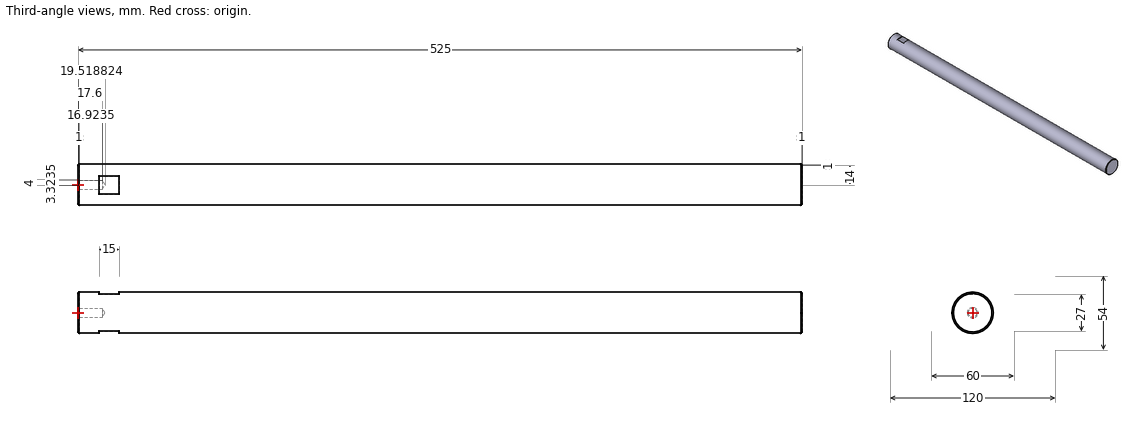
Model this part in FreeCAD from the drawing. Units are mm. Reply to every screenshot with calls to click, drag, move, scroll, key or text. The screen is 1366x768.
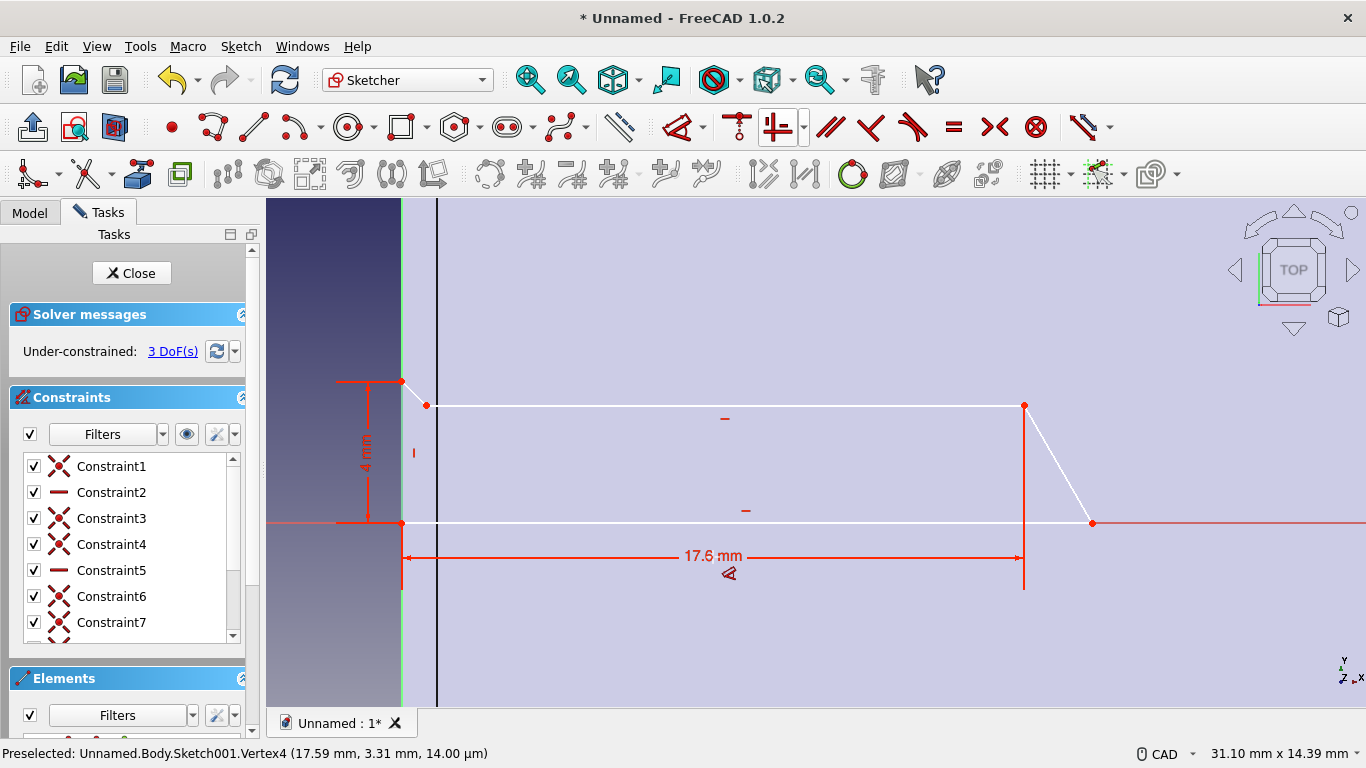
click(845, 406)
click(725, 372)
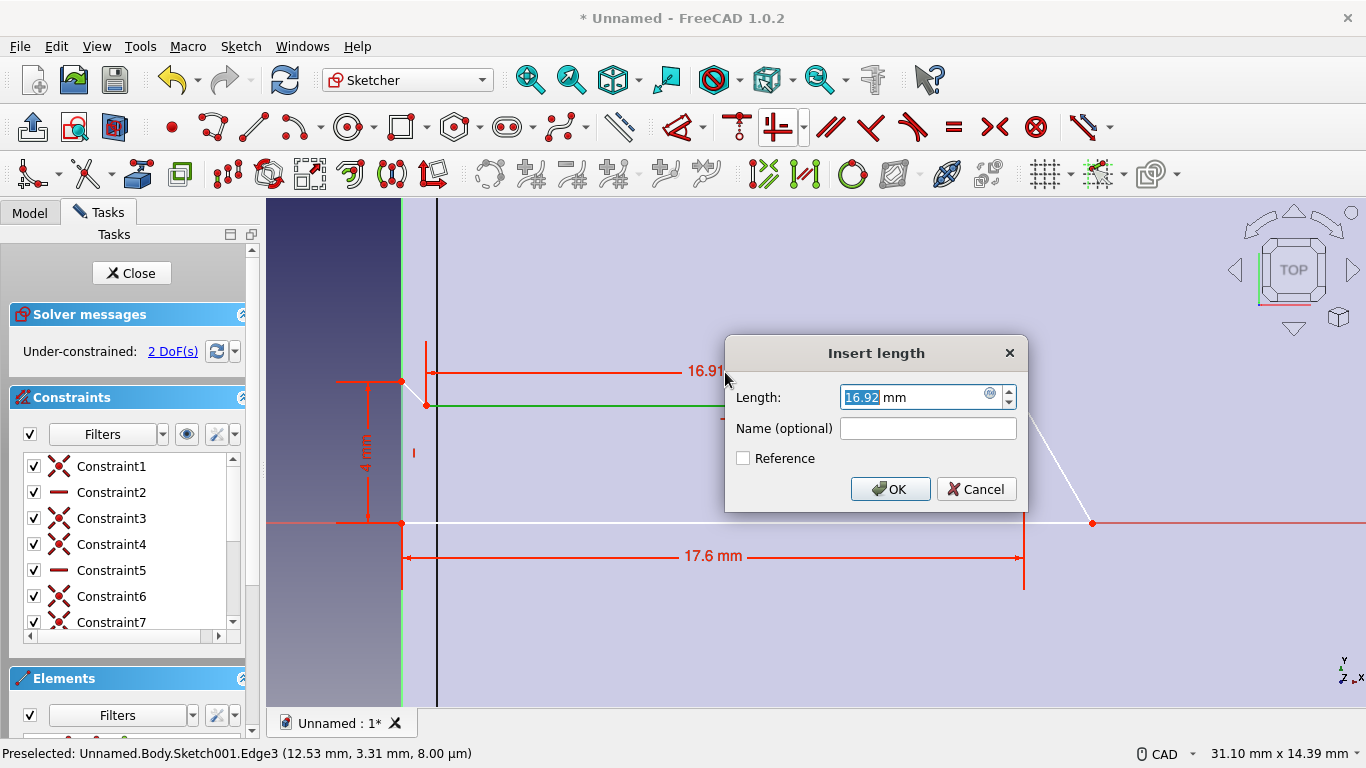
text(16.9235)
key(Return)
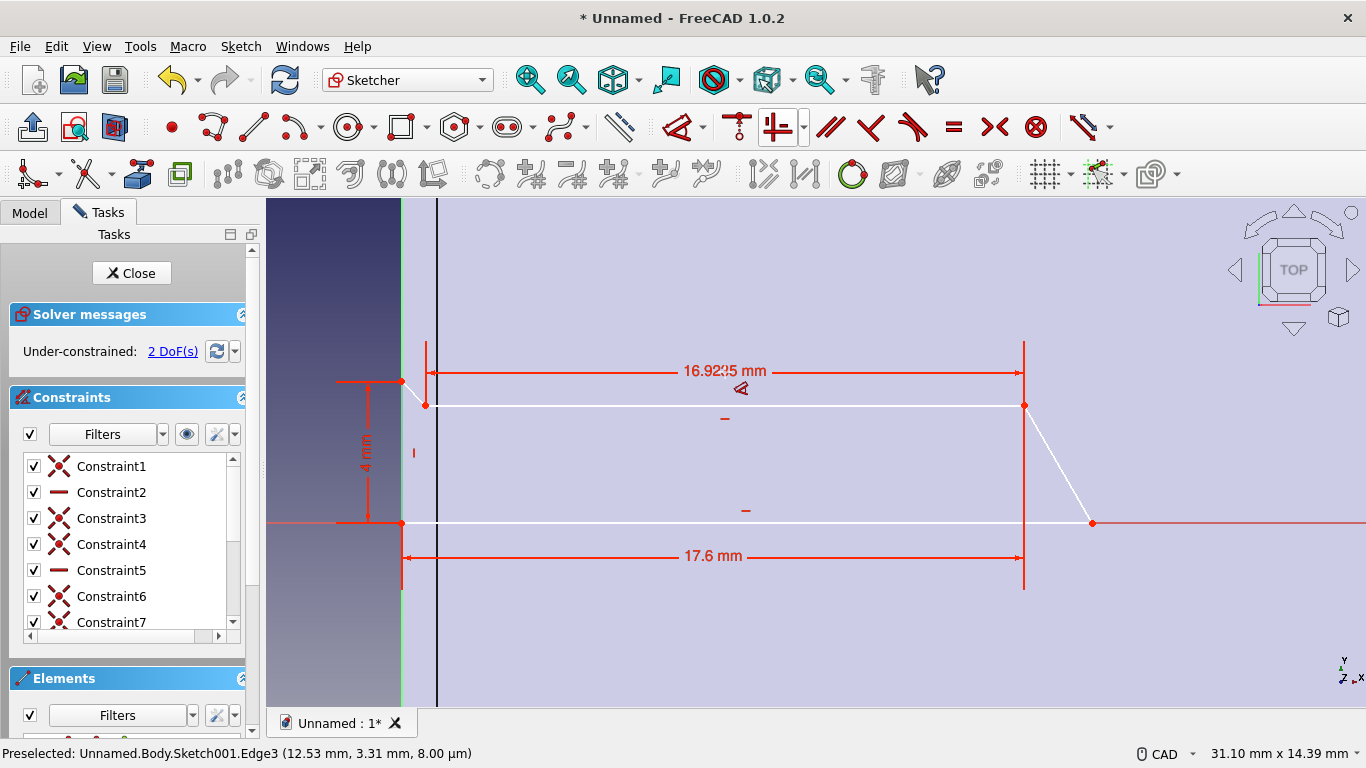
click(1024, 406)
click(368, 491)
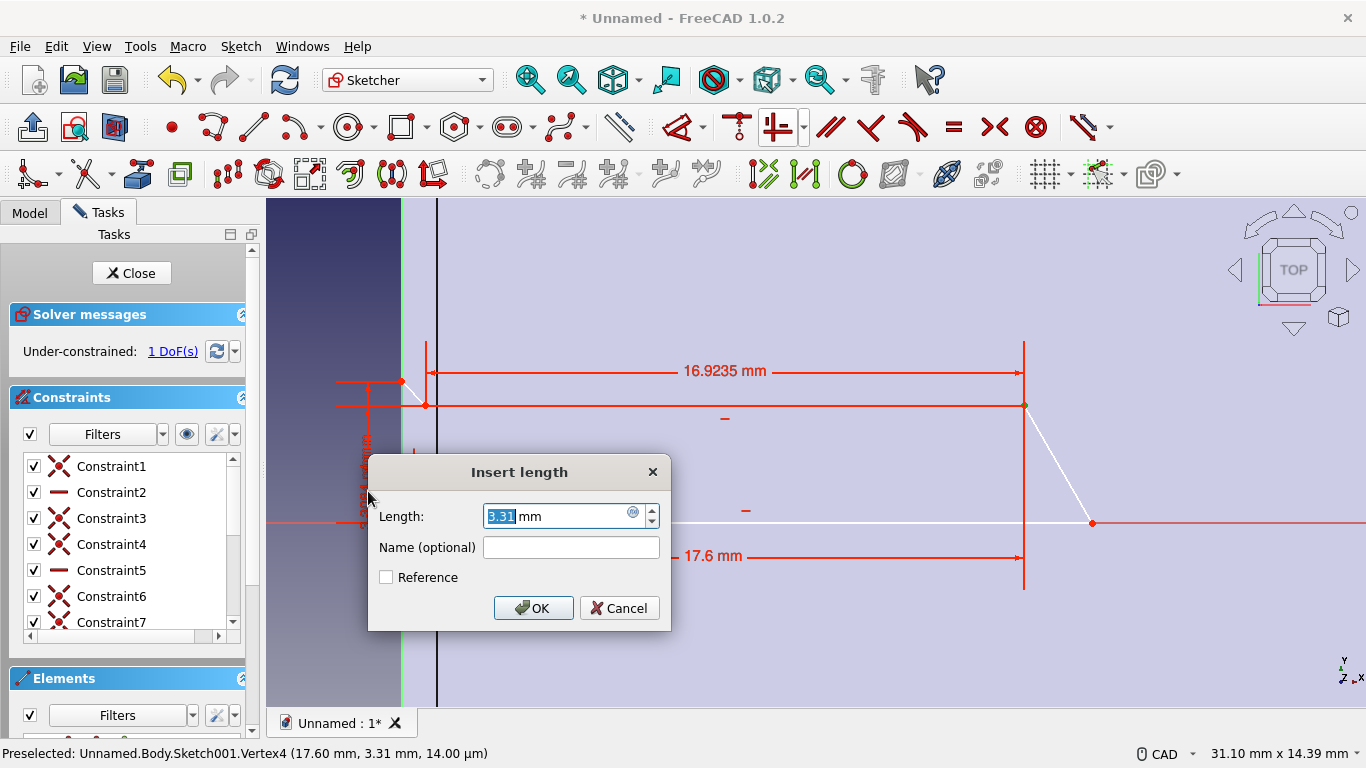
text(3.3235)
key(Return)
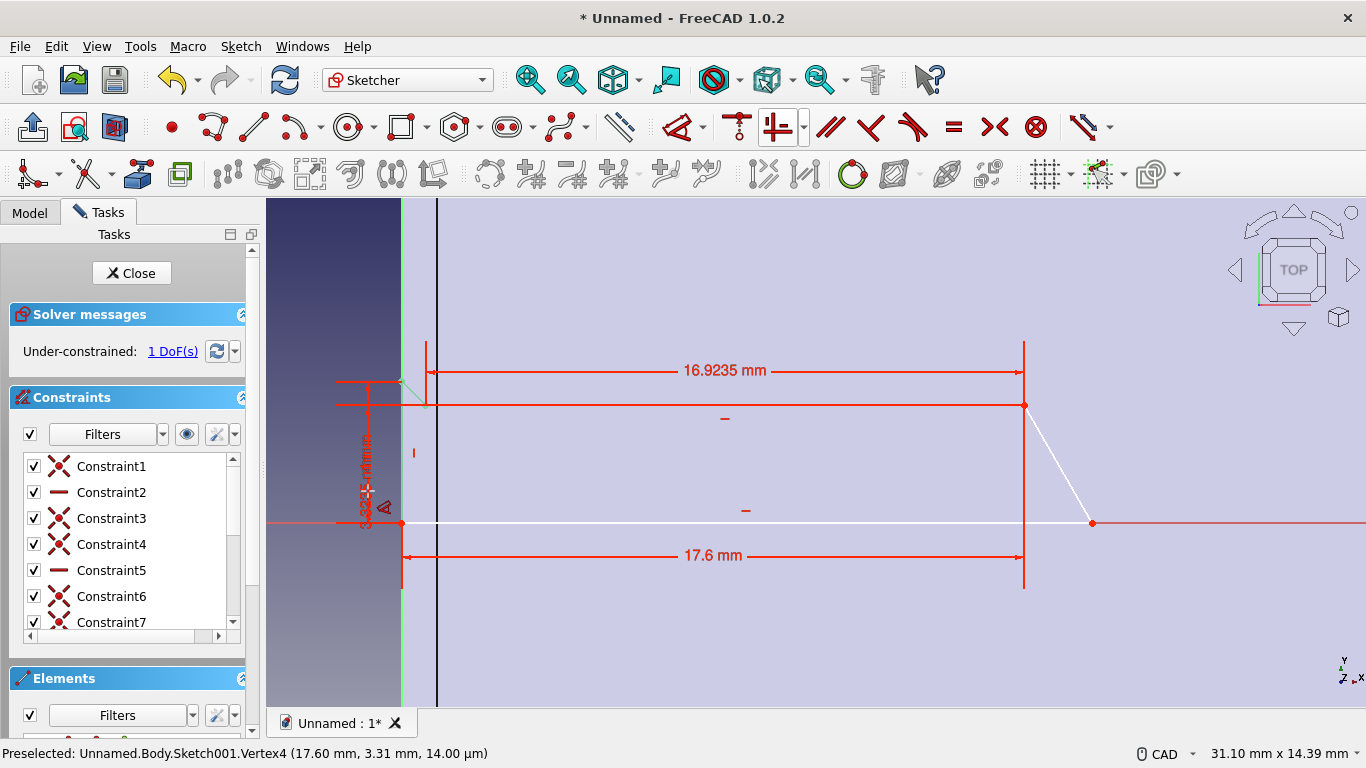
click(609, 523)
click(588, 557)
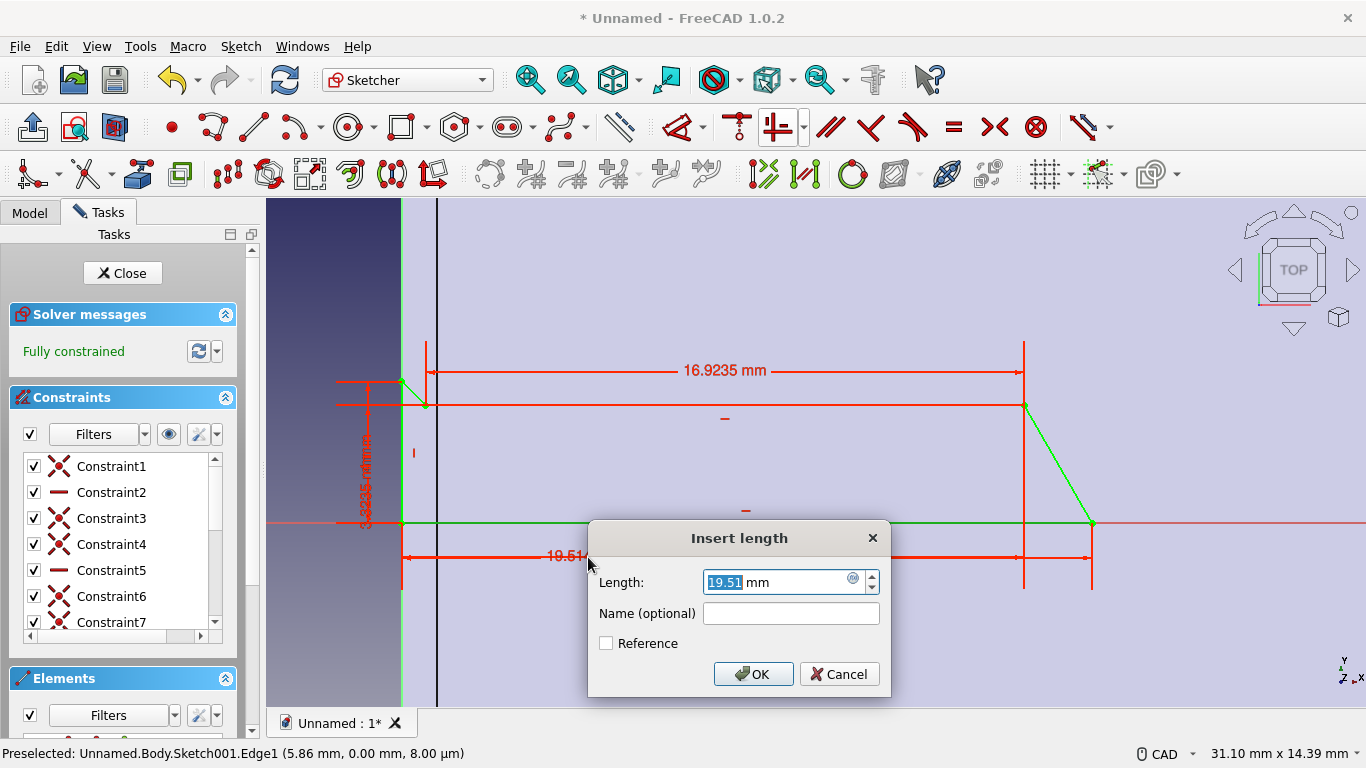
text(19.518824)
key(Return)
key(Escape)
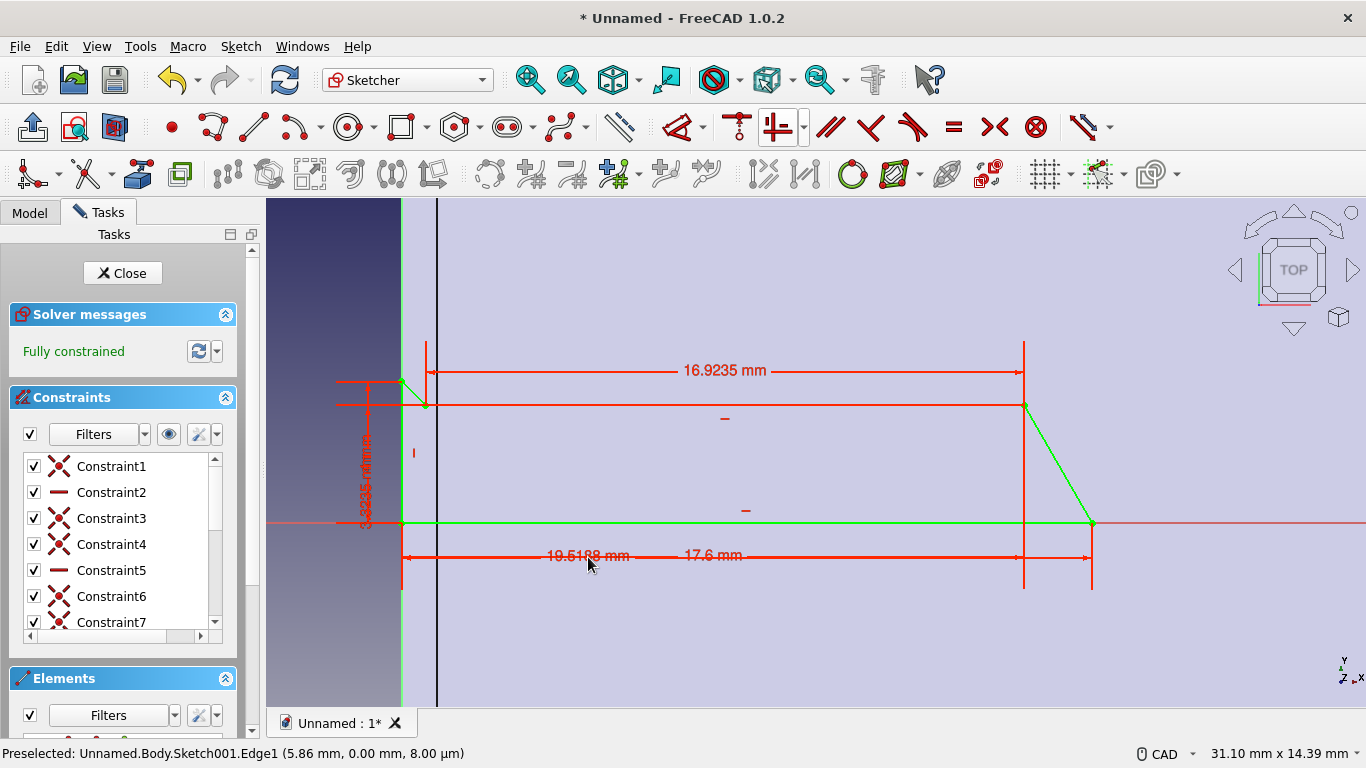
click(123, 273)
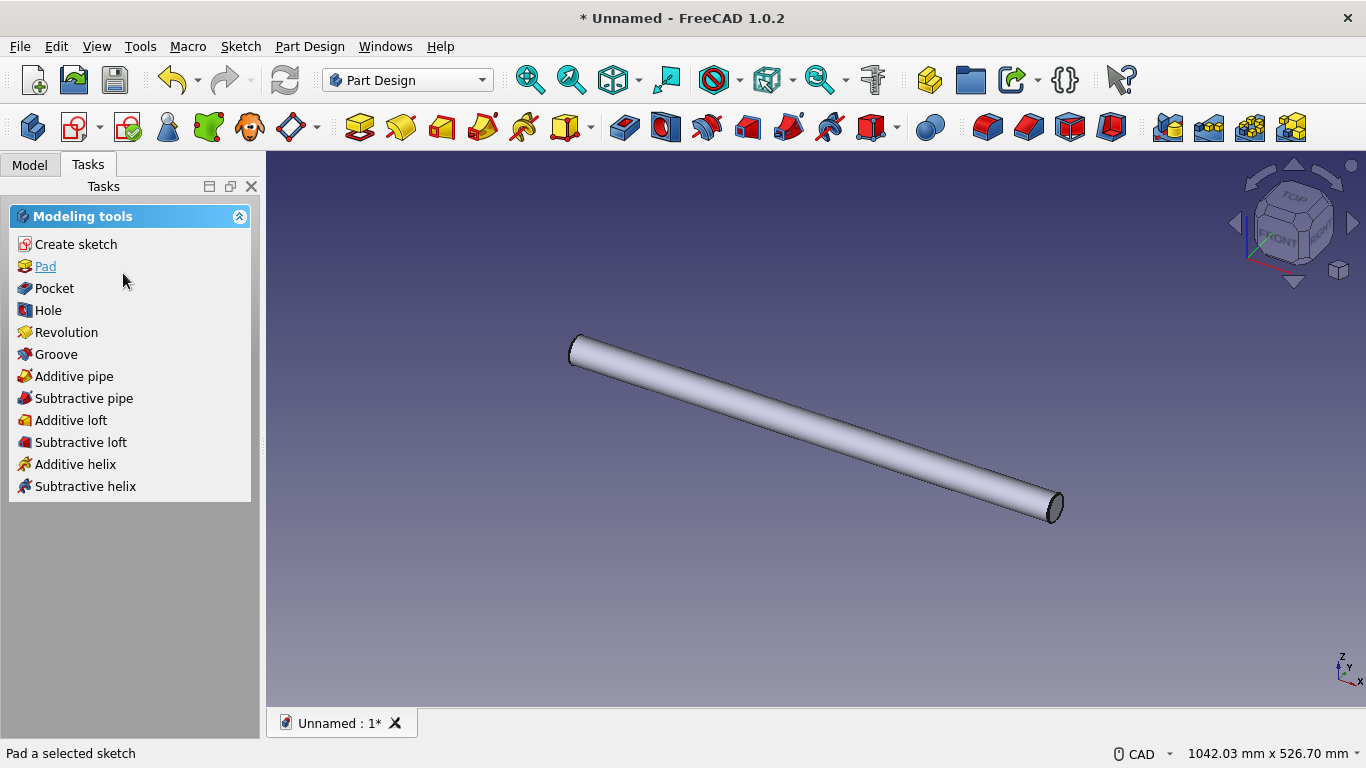
click(707, 128)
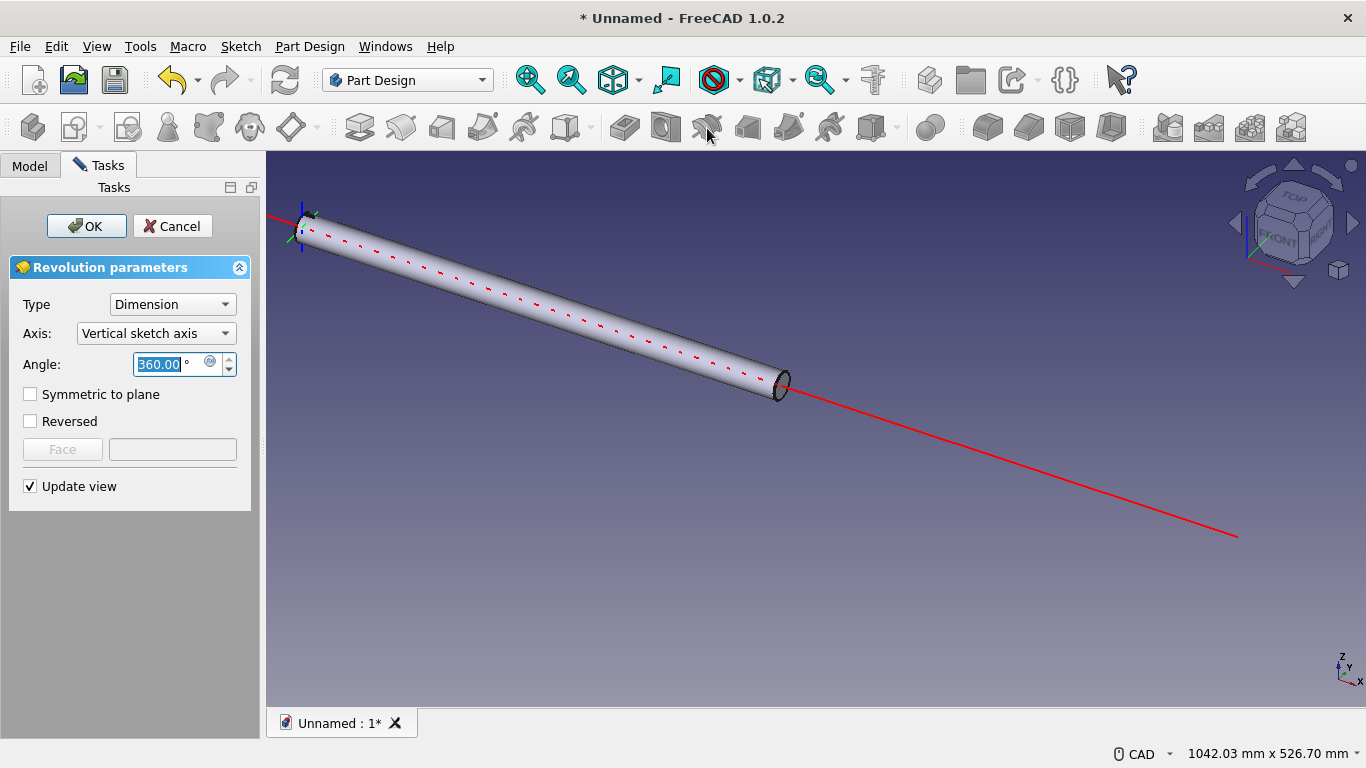
click(157, 334)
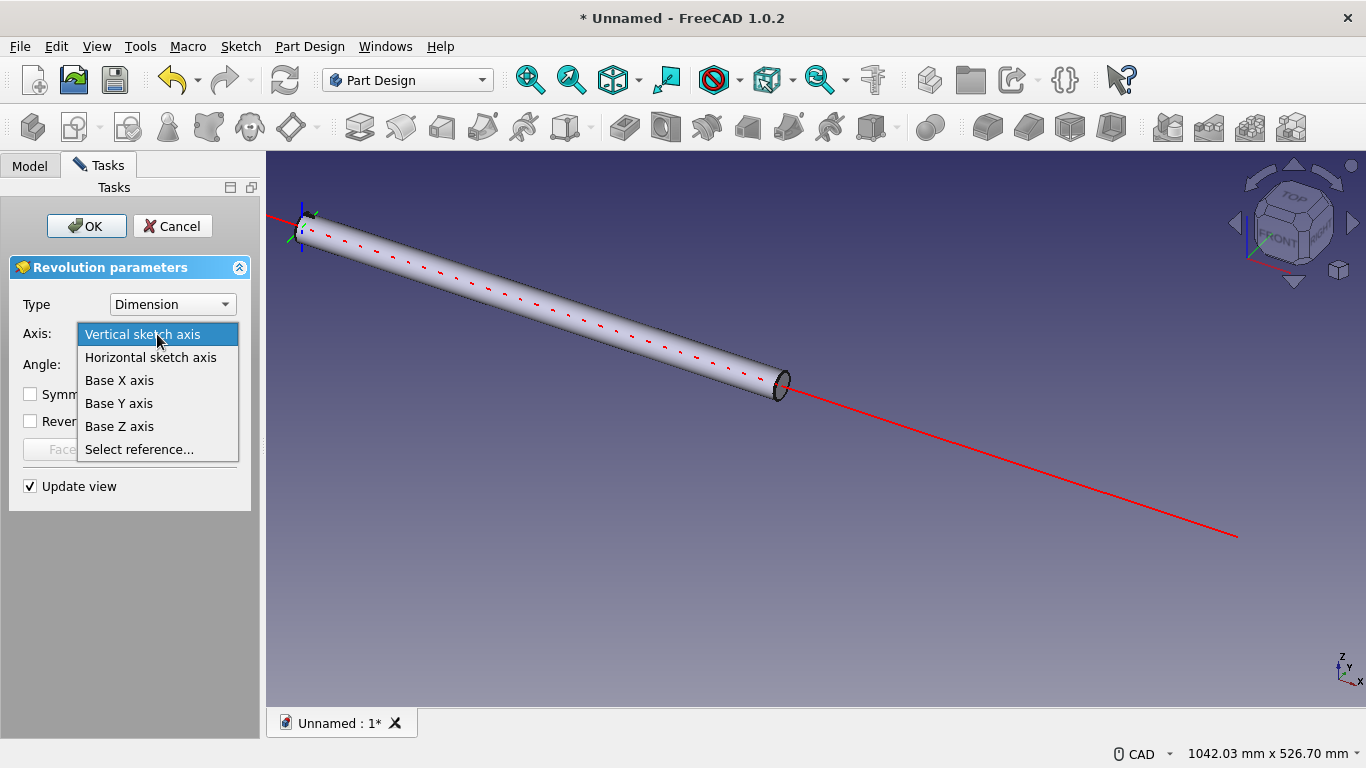
click(156, 358)